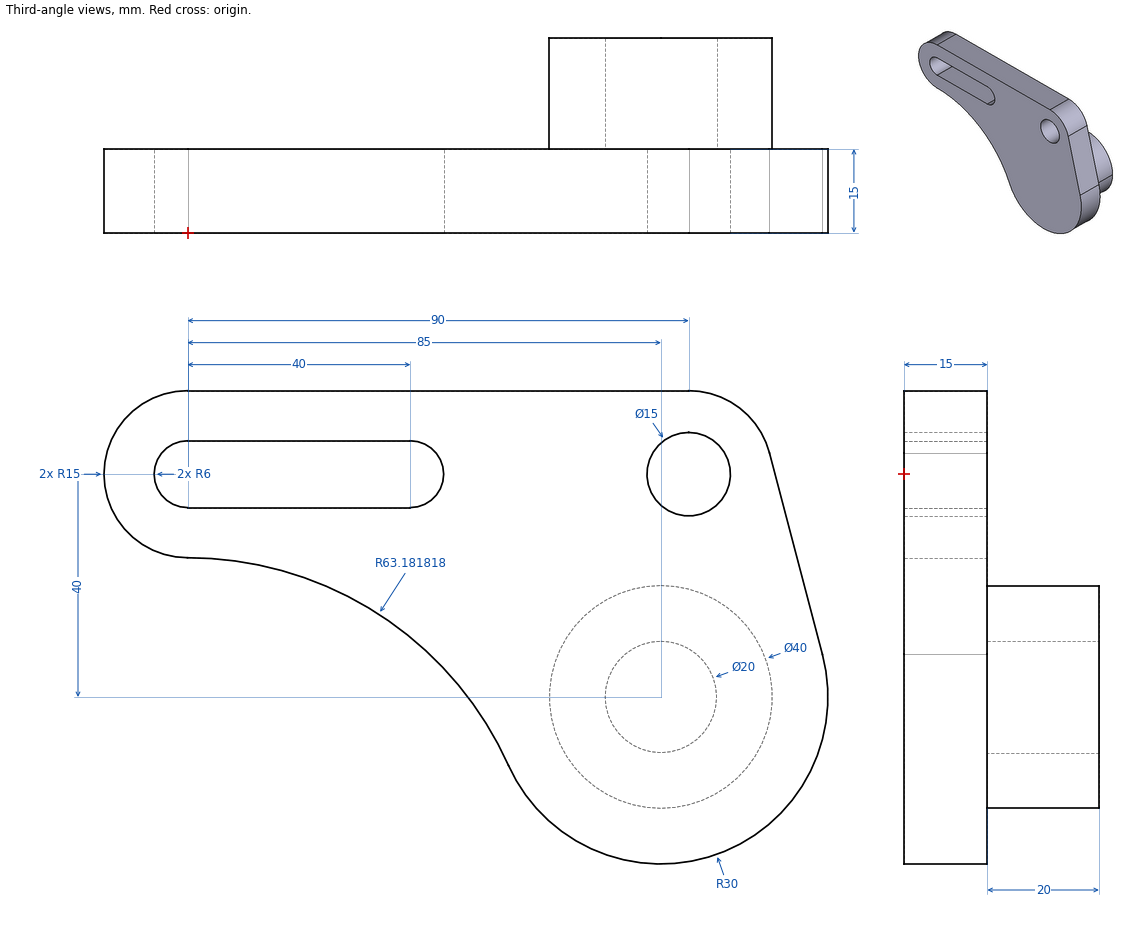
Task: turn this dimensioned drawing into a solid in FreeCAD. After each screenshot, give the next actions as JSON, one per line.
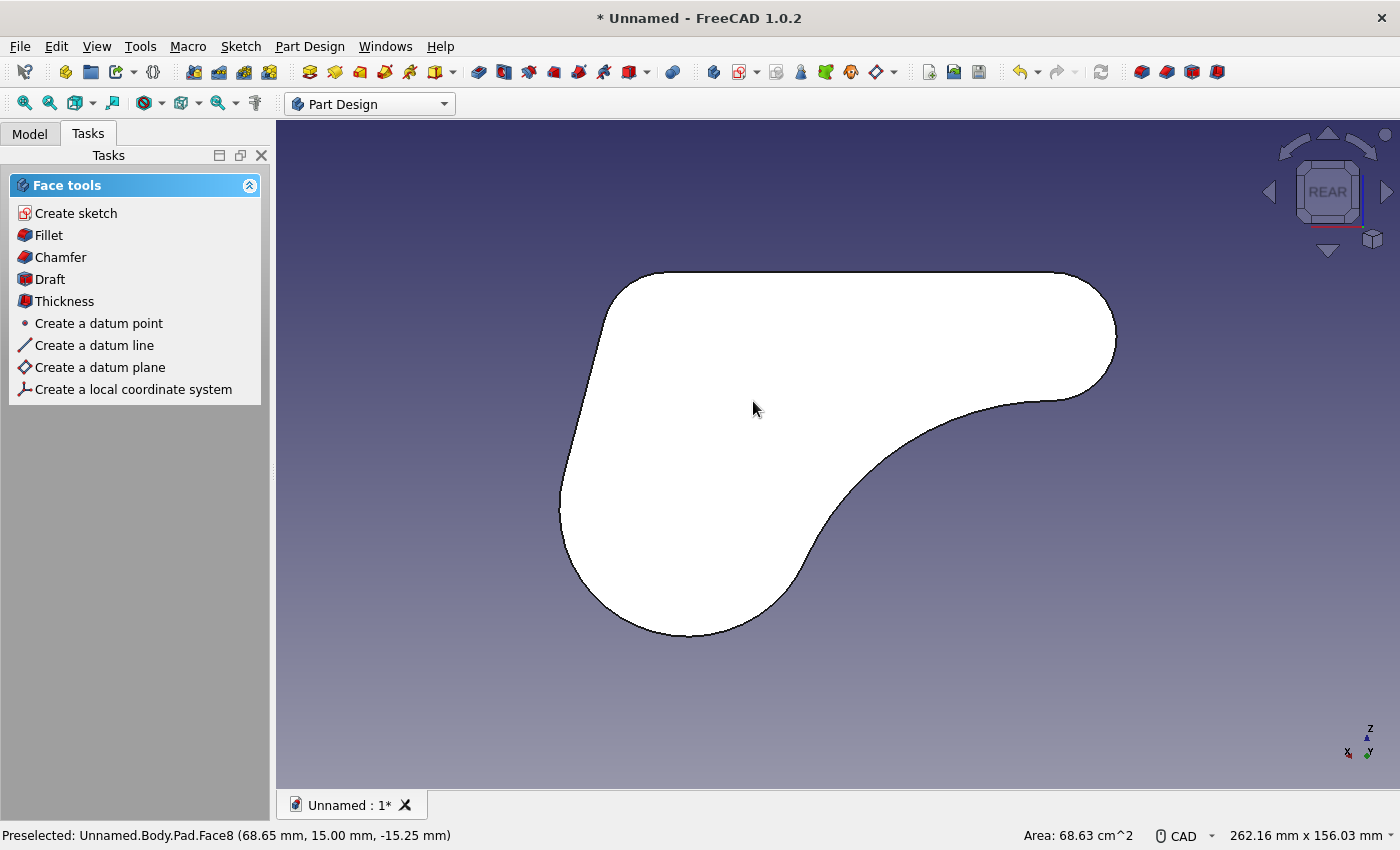
{"action": "left_click", "coordinate": [738, 72]}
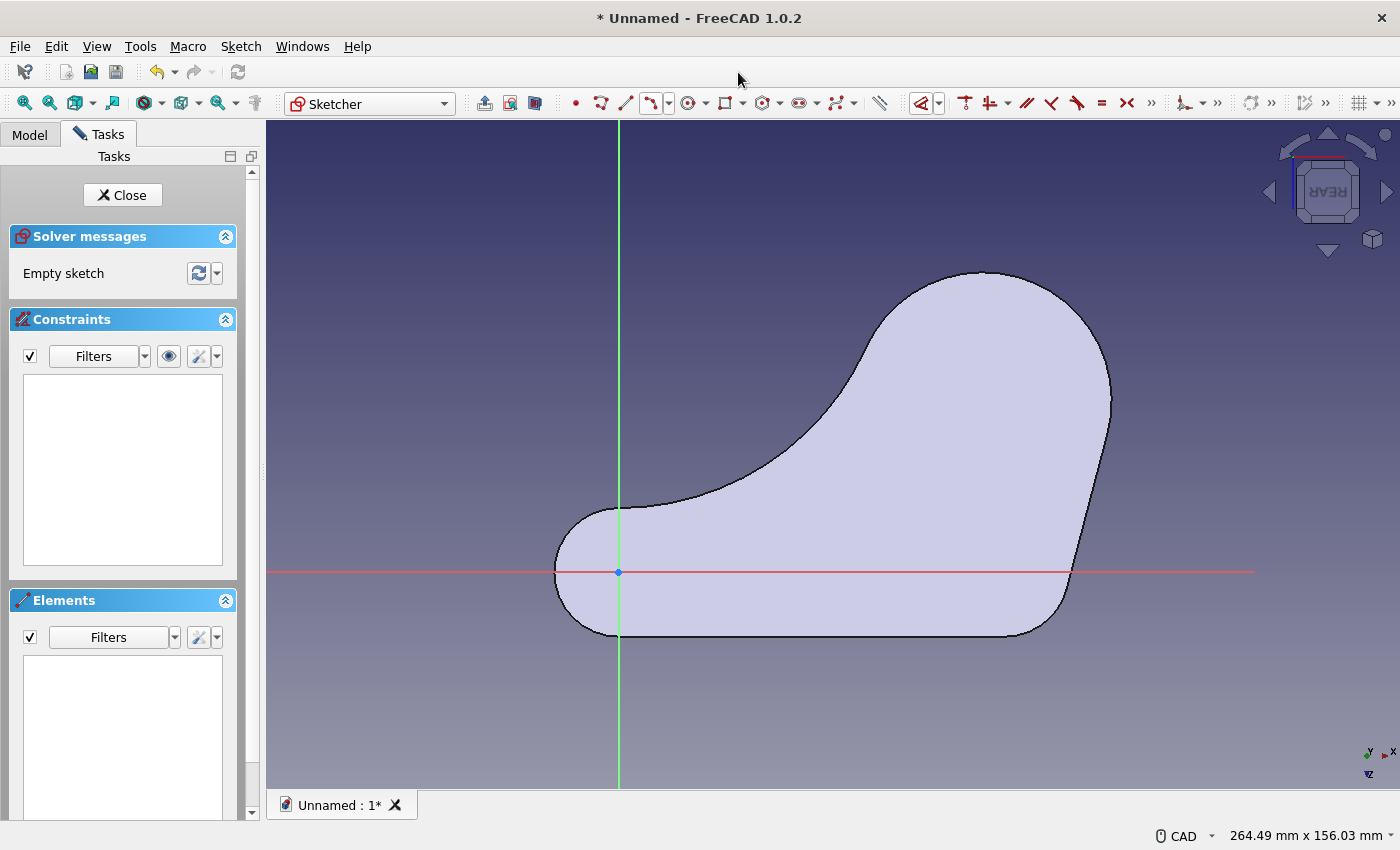
{"action": "scroll", "coordinate": [669, 641], "scroll_direction": "up", "scroll_amount": 5}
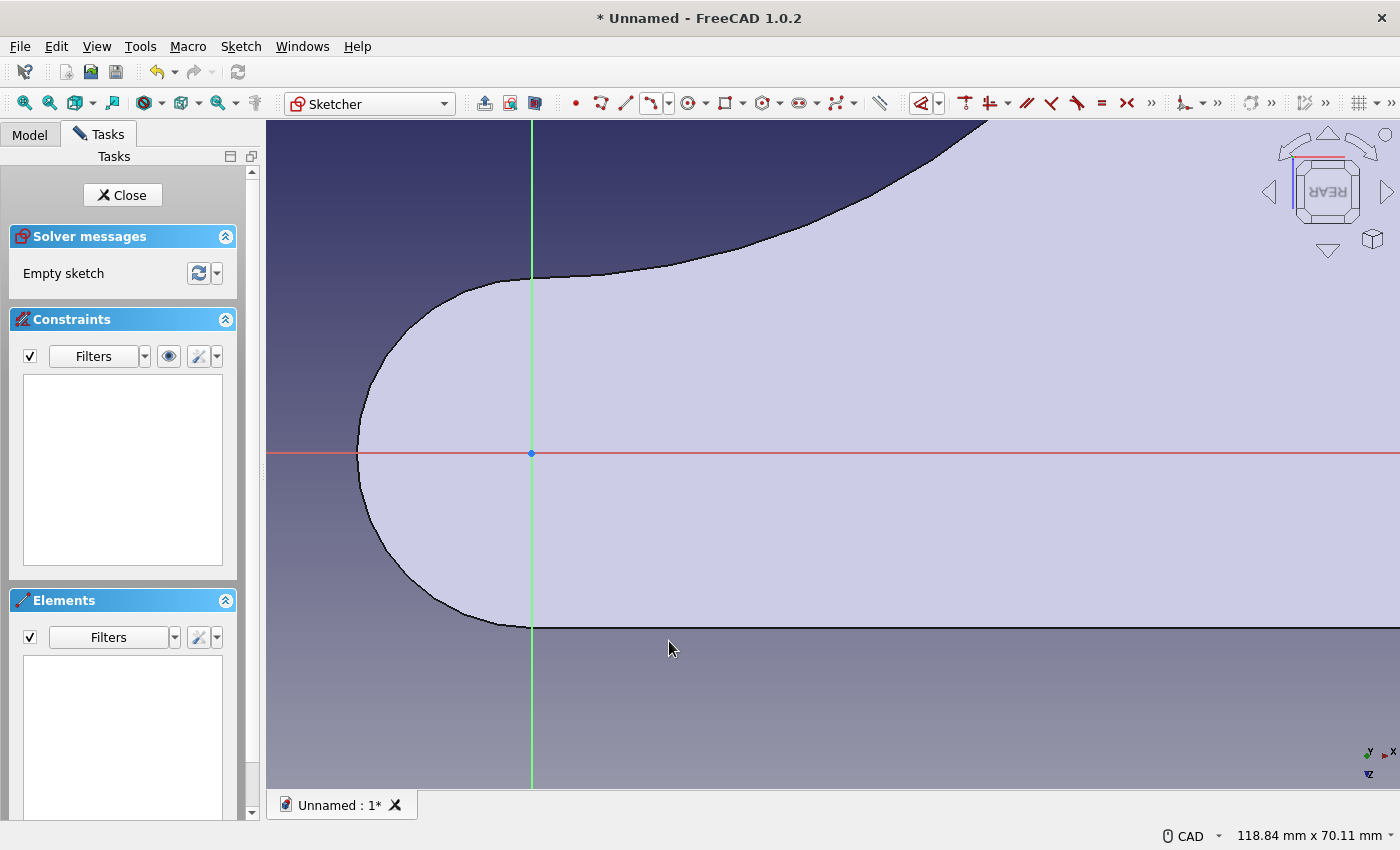
{"action": "left_click", "coordinate": [798, 104]}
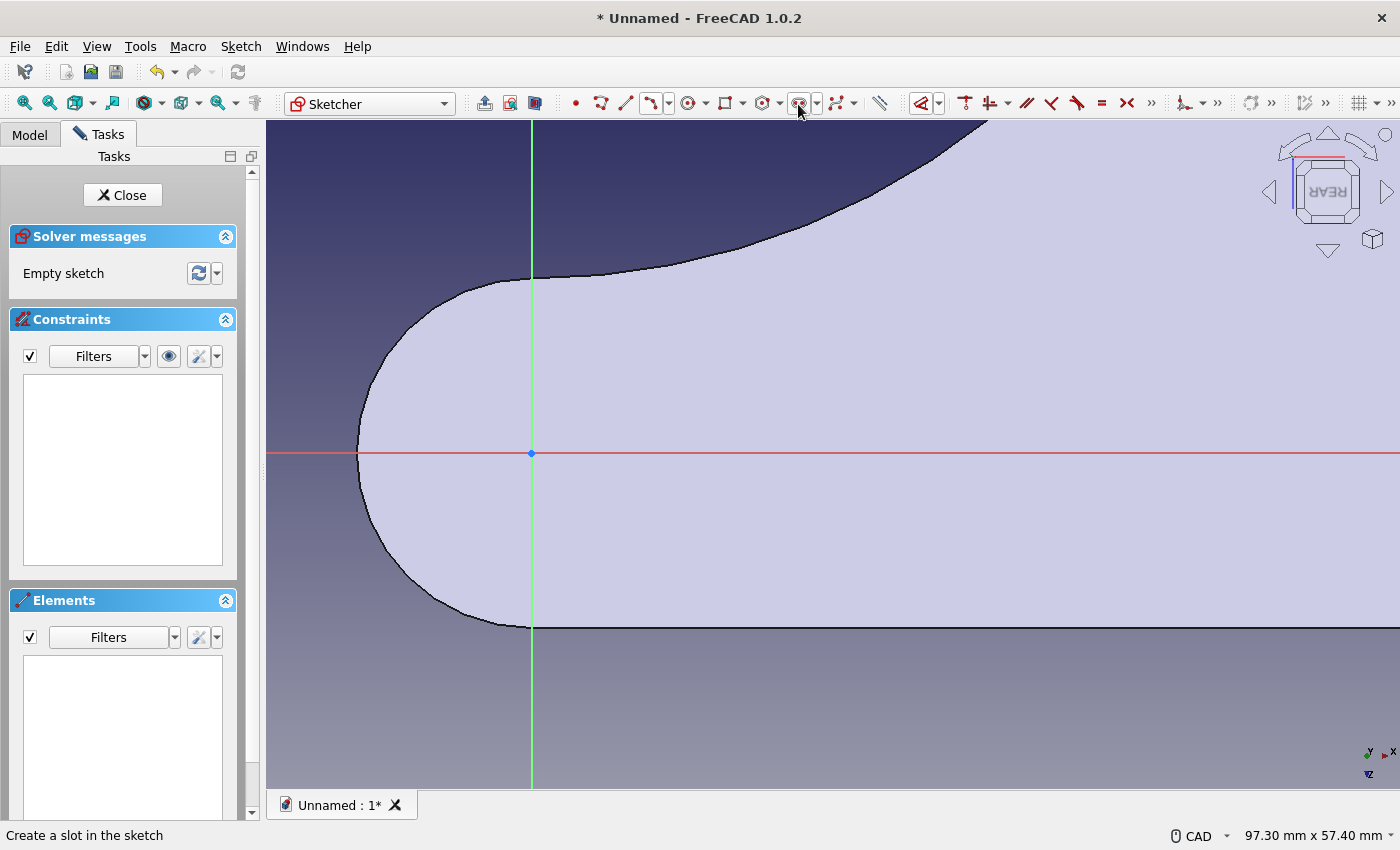
{"action": "left_click", "coordinate": [532, 453]}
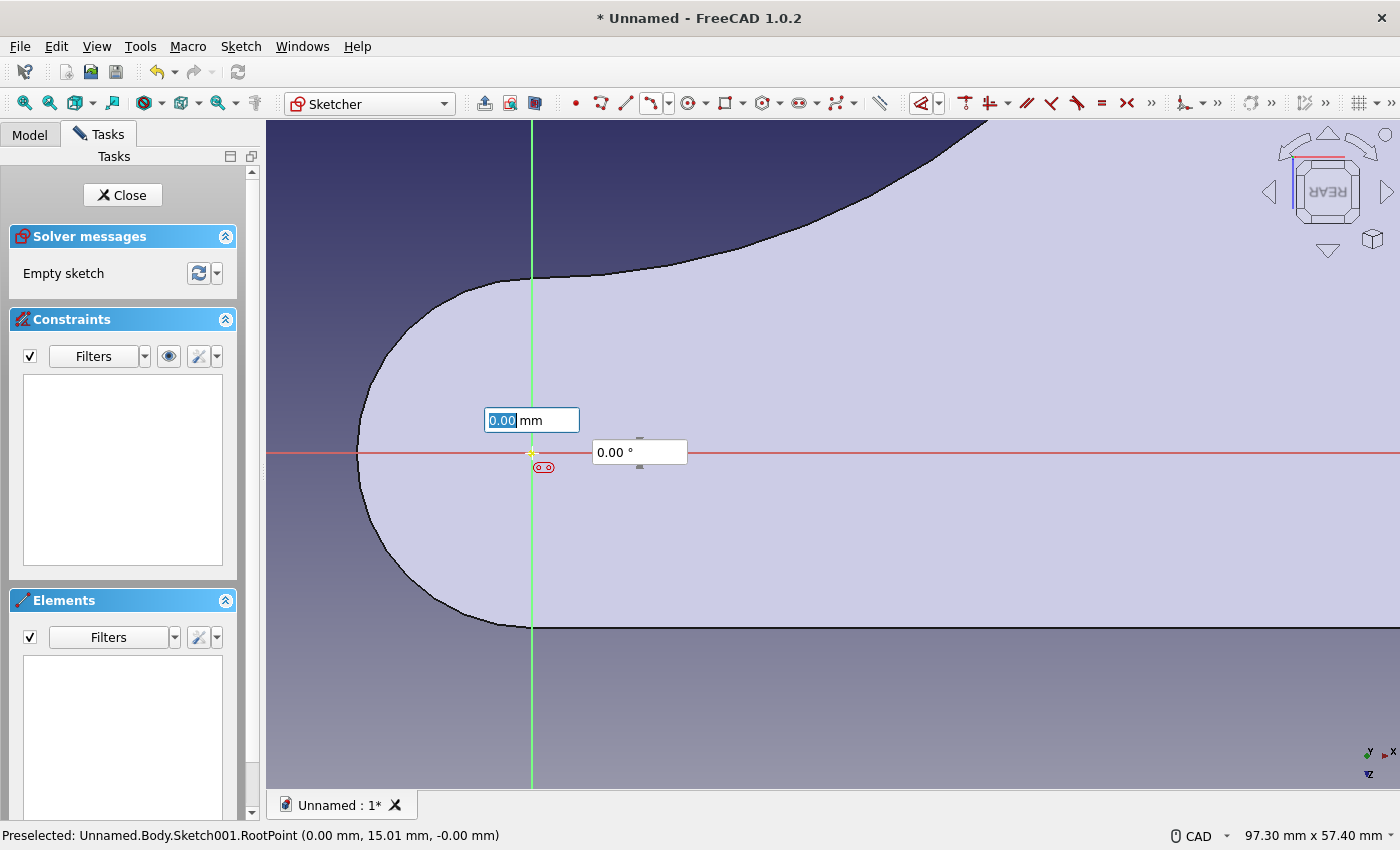
{"action": "left_click", "coordinate": [998, 444]}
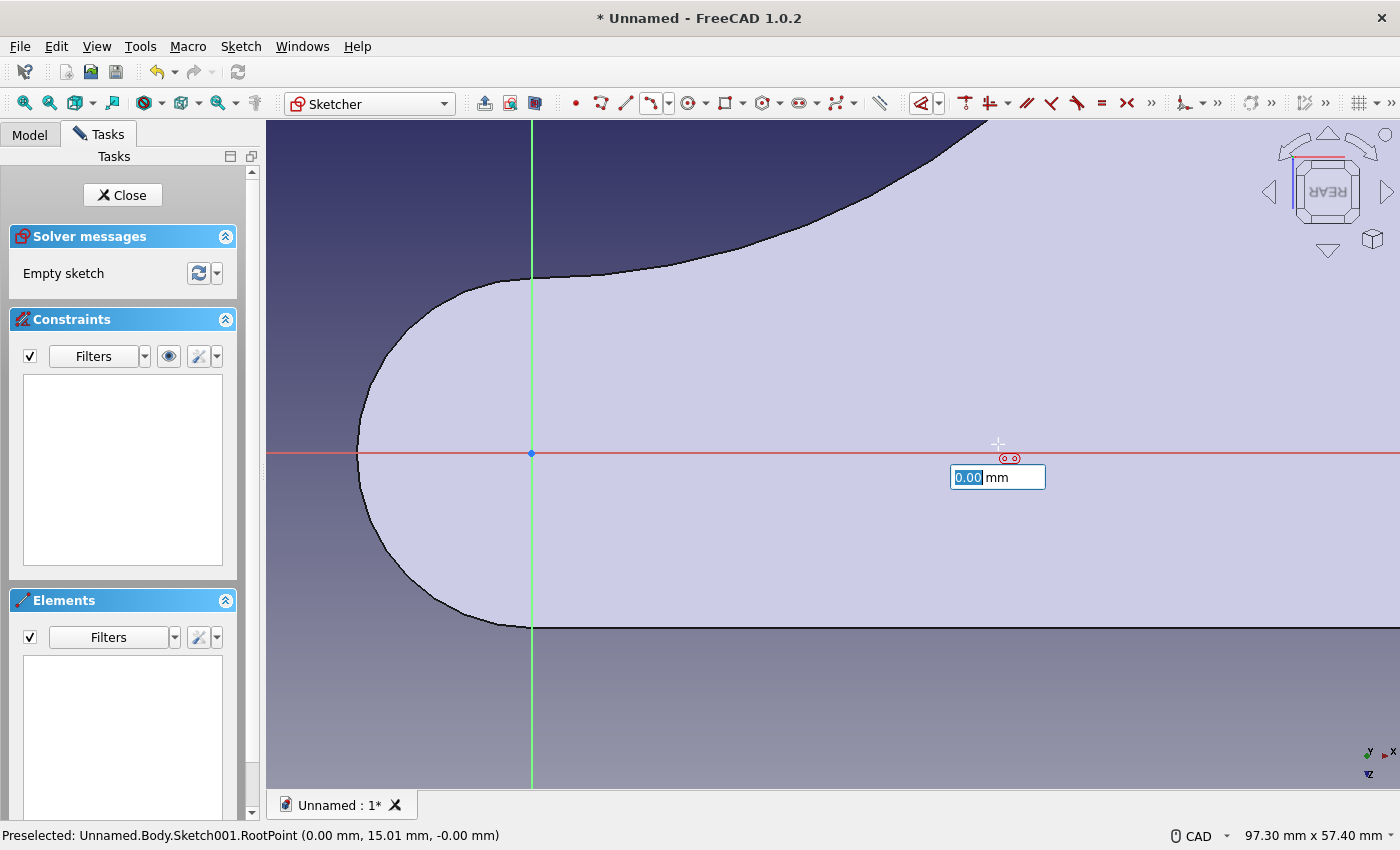
{"action": "left_click", "coordinate": [765, 383]}
{"action": "key", "text": "Escape"}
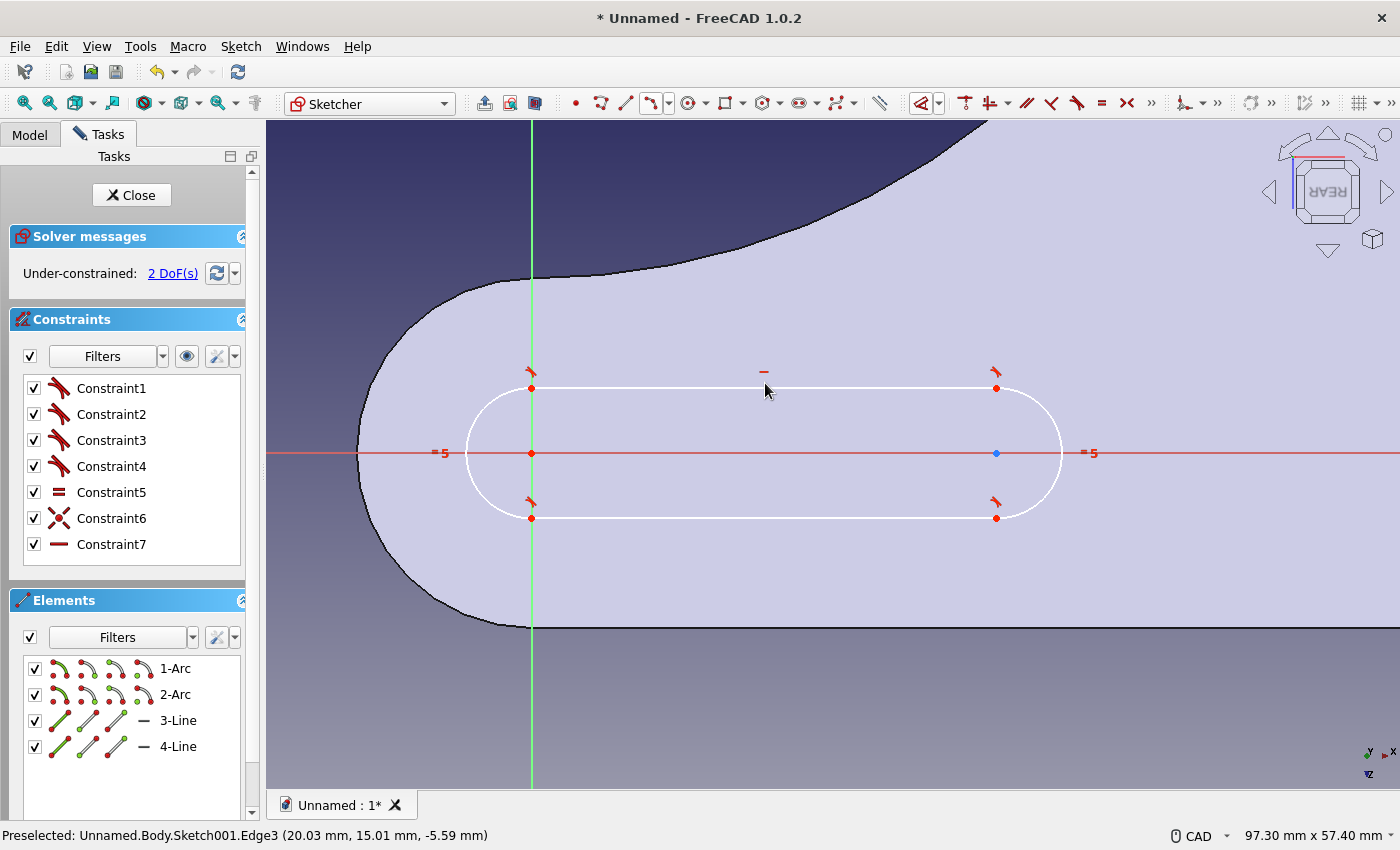
{"action": "left_click", "coordinate": [479, 415]}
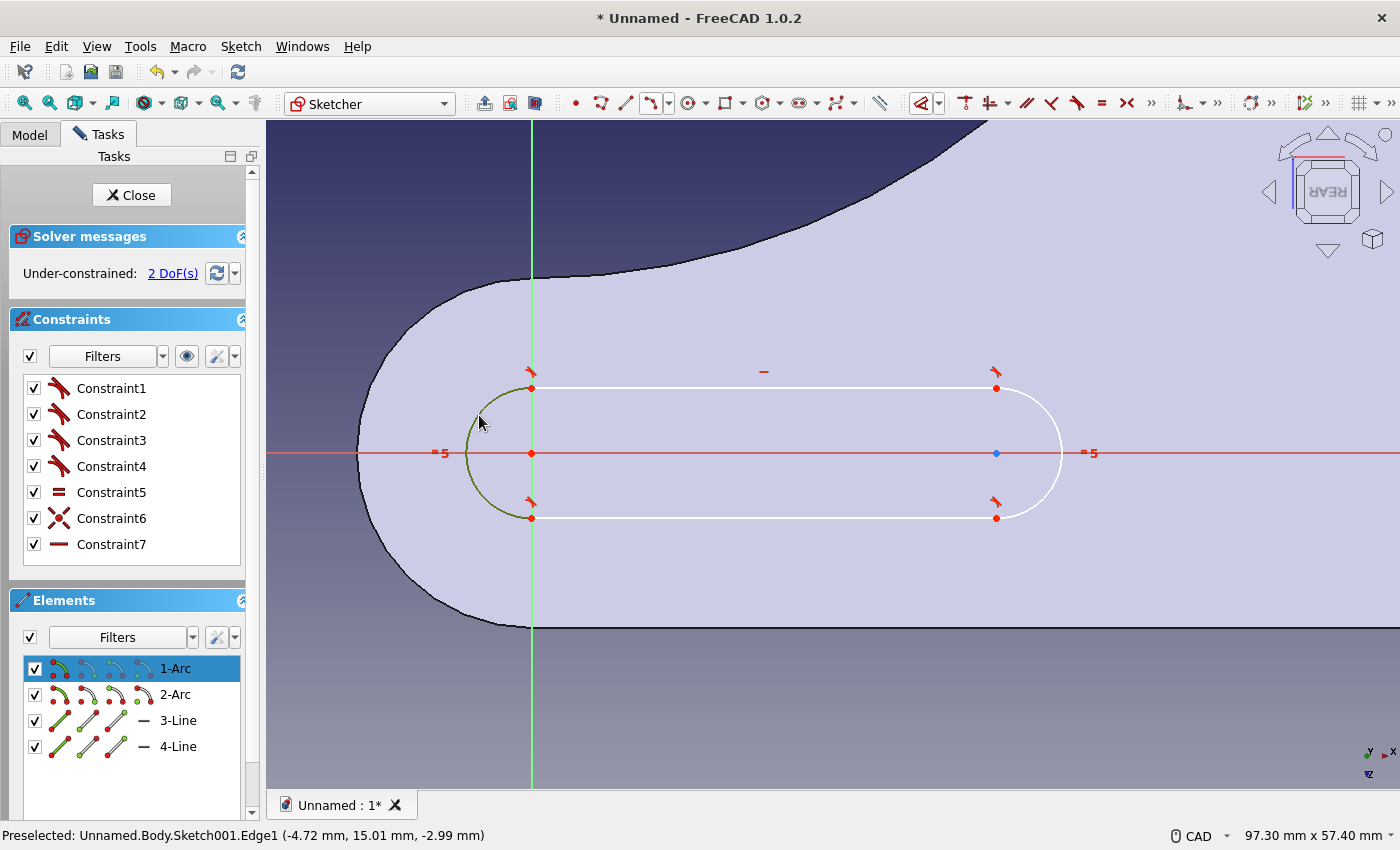
{"action": "key", "text": "k r"}